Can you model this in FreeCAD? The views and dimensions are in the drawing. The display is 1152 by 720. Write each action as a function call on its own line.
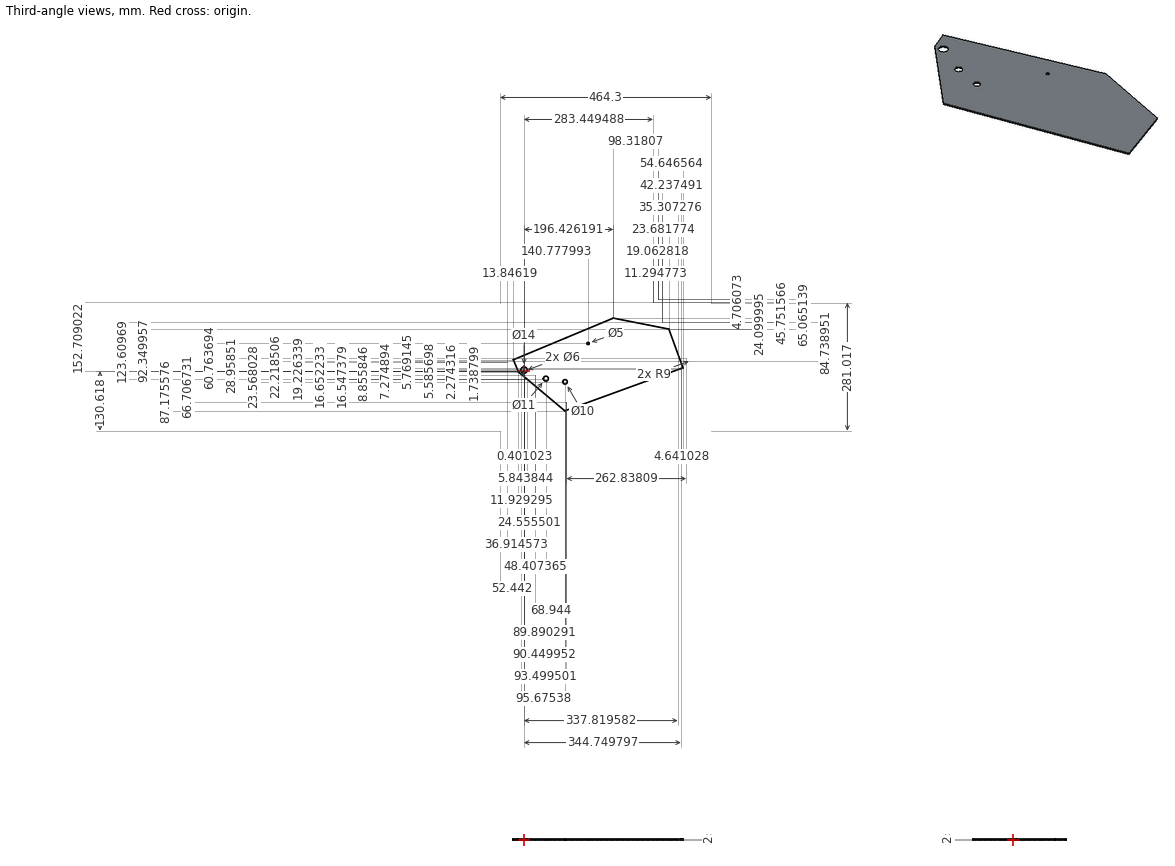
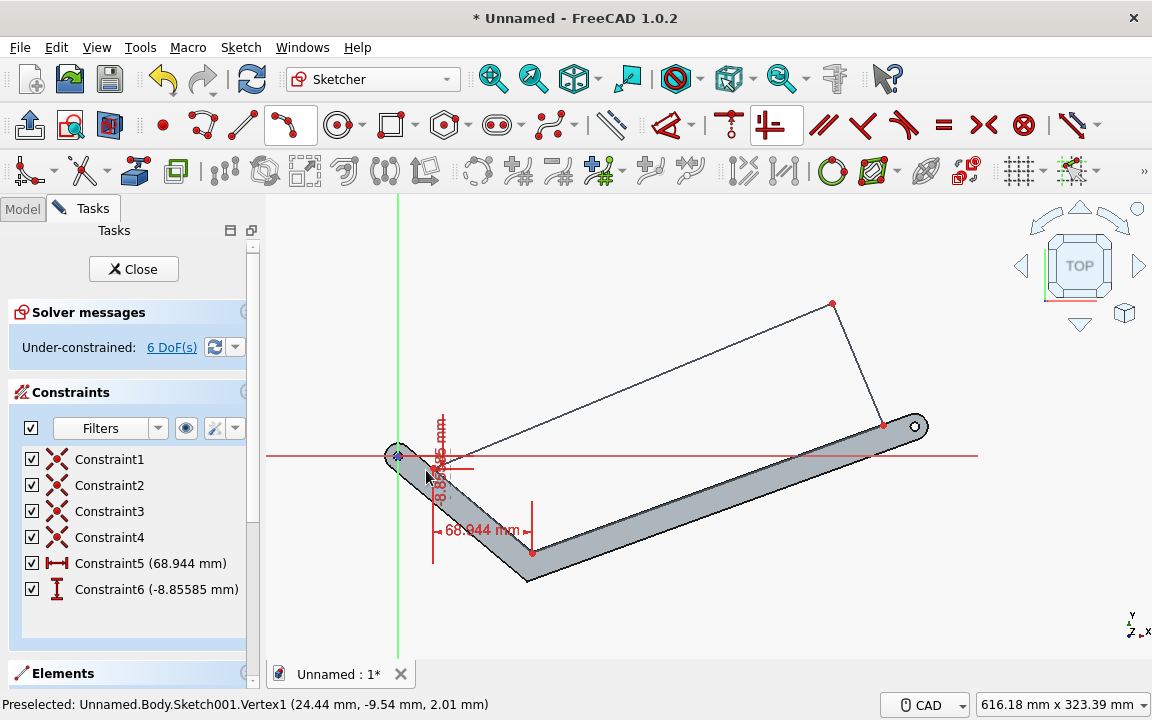
click(433, 469)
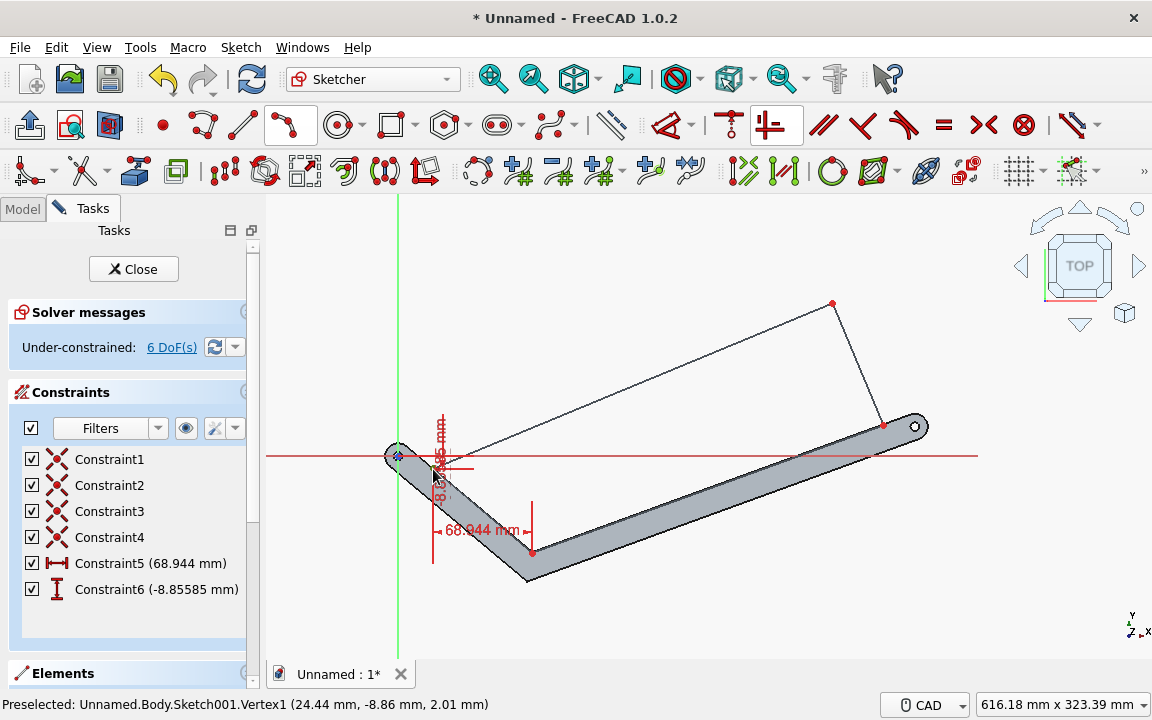
key(l)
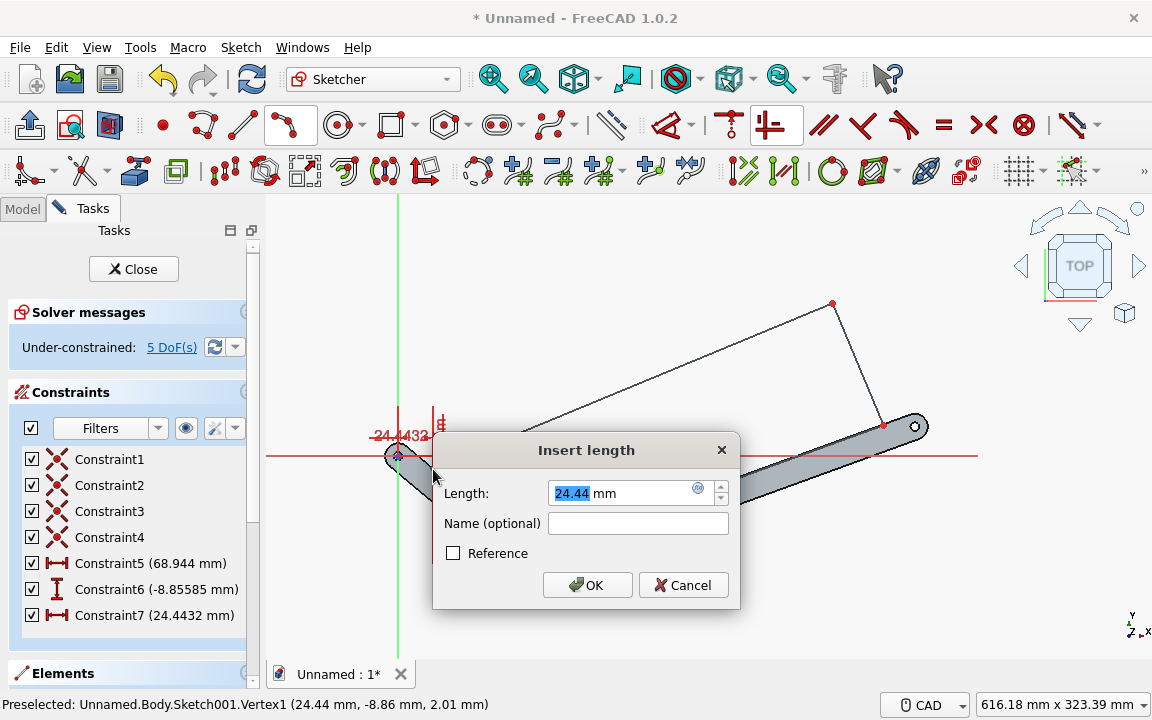
text(24.555501)
key(Return)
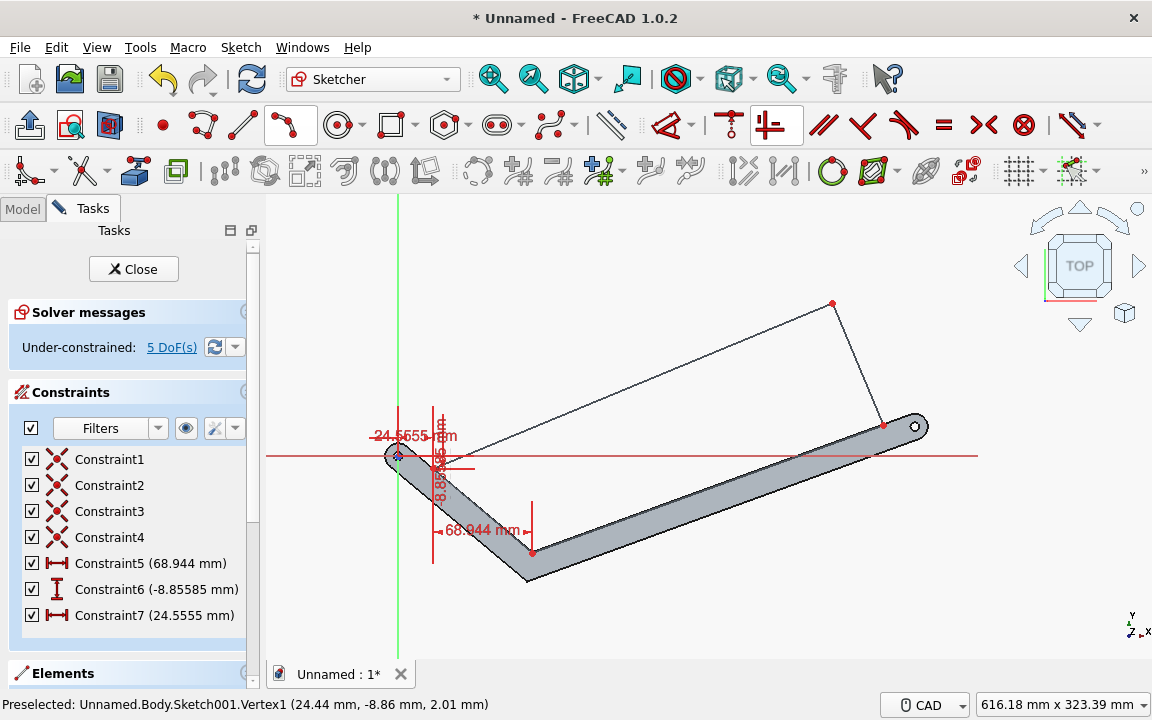
click(532, 553)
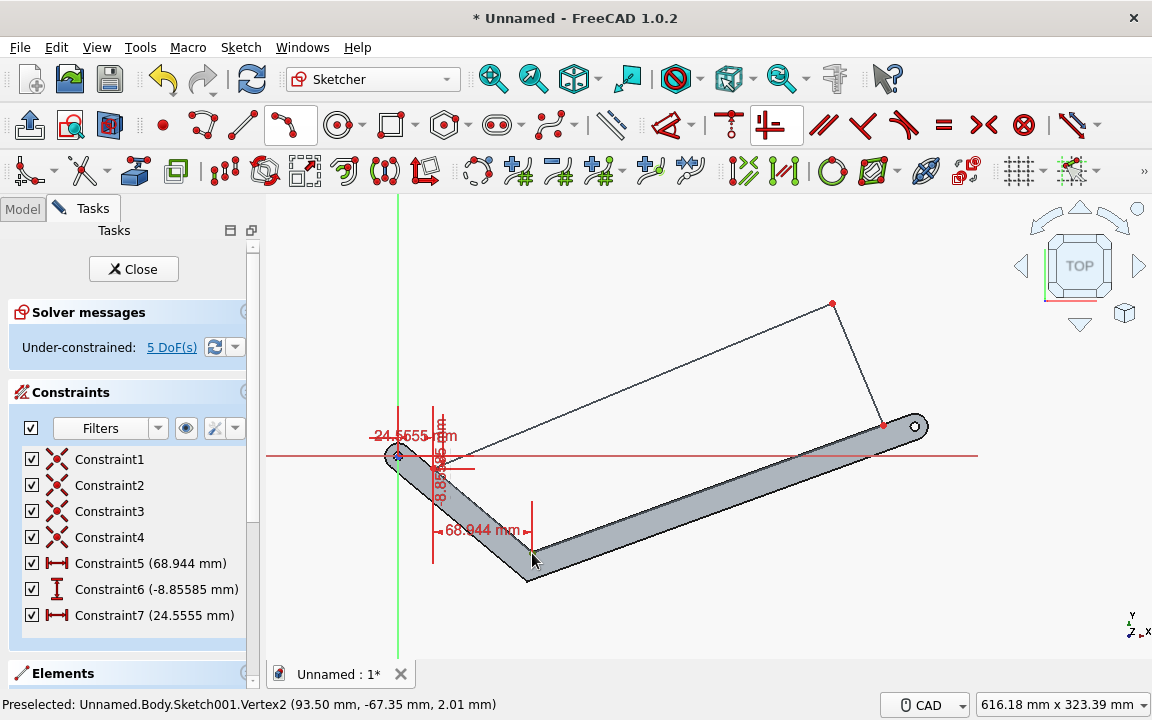
key(i)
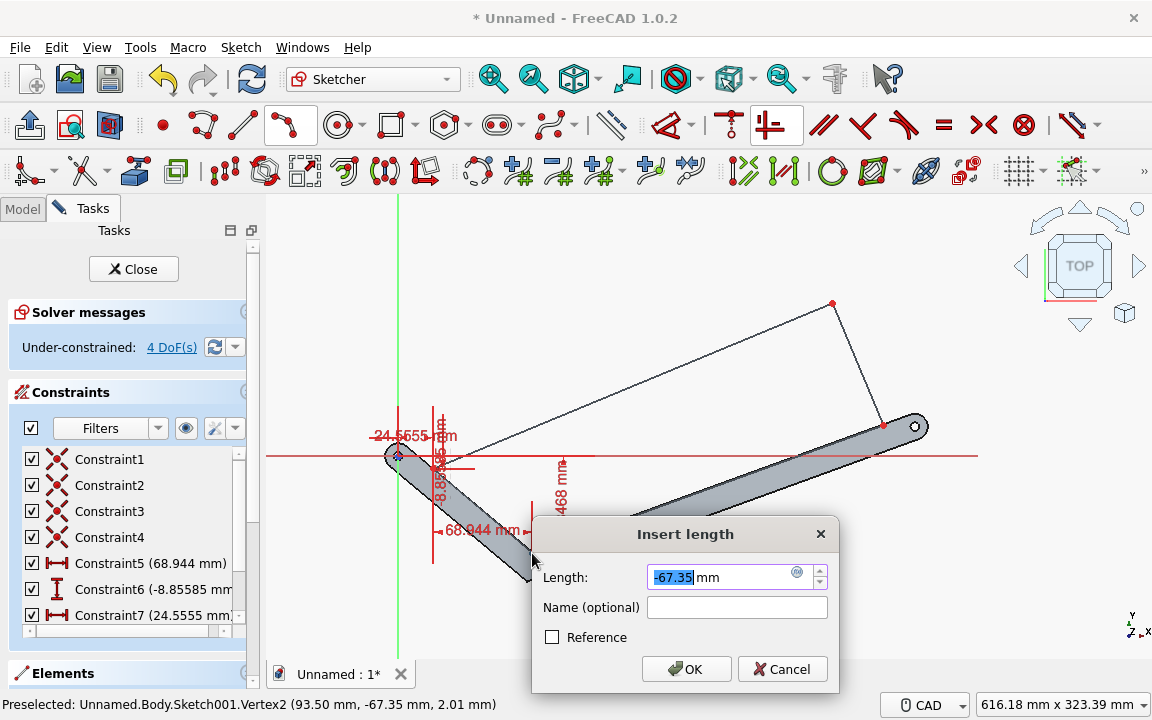
text(-66.706731)
key(Return)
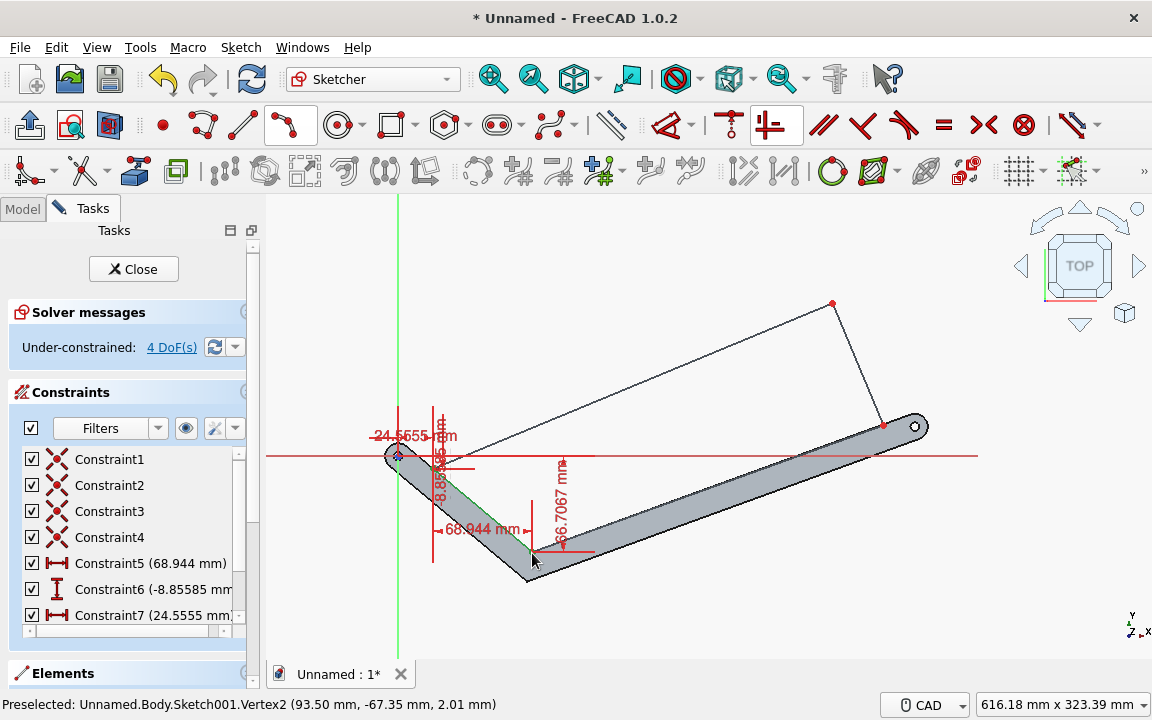
scroll(884, 425, up, 2)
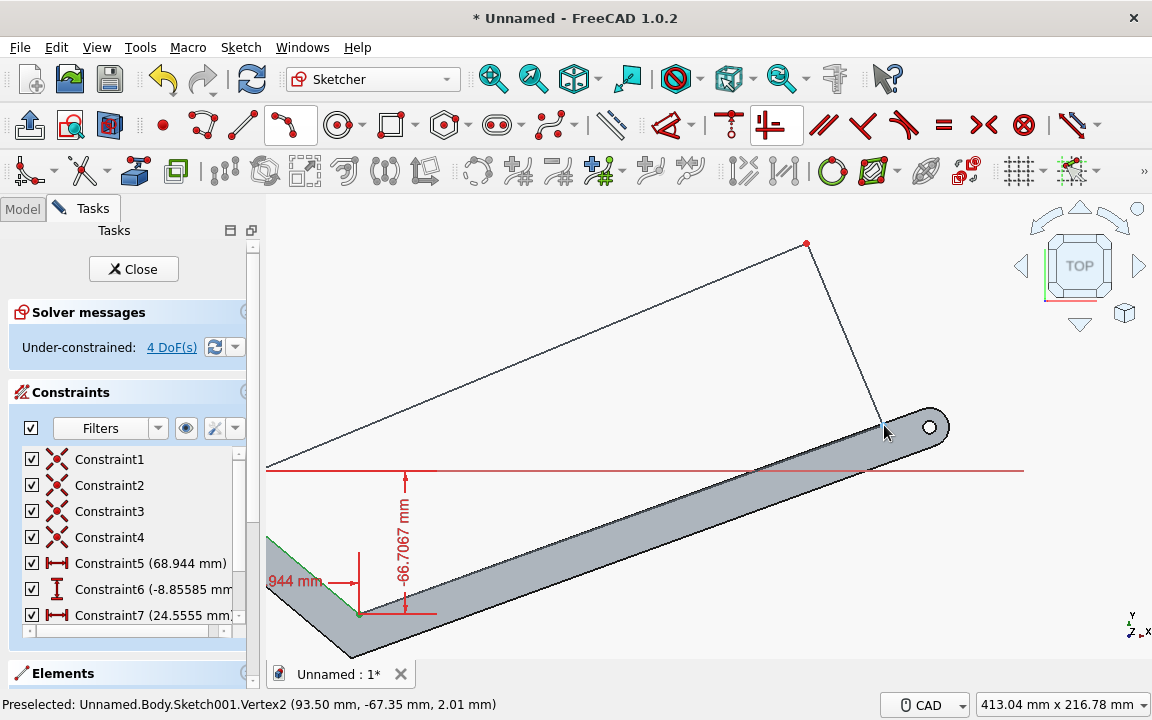
click(883, 425)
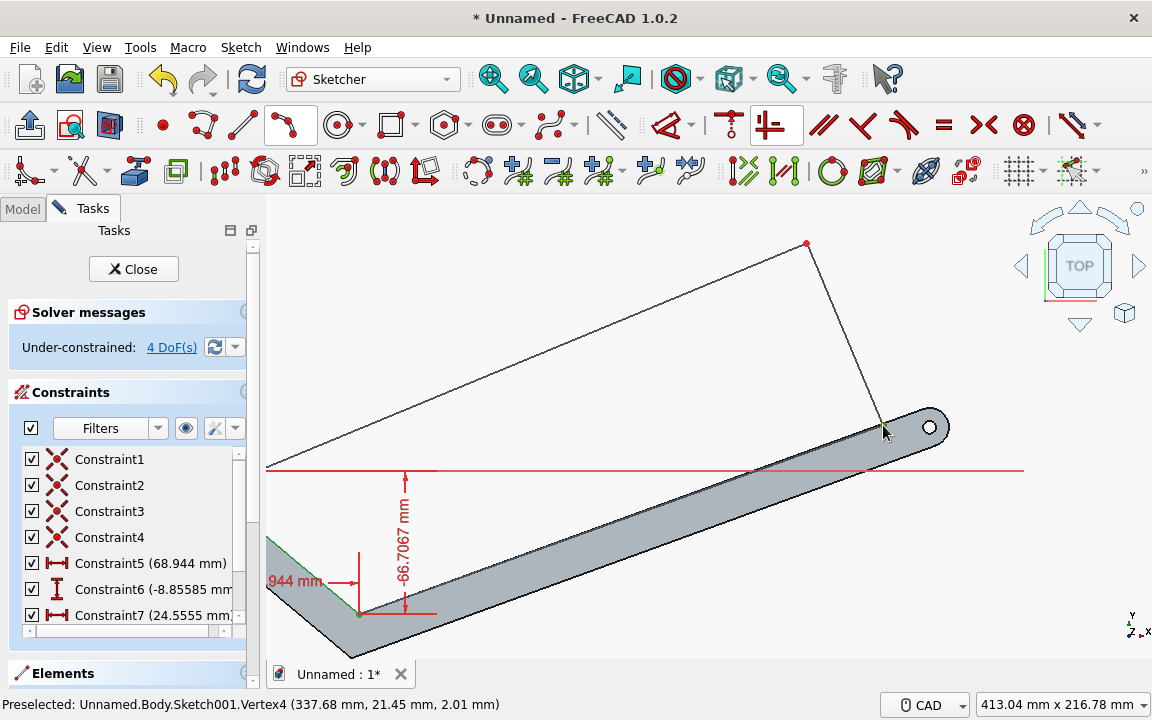
key(i)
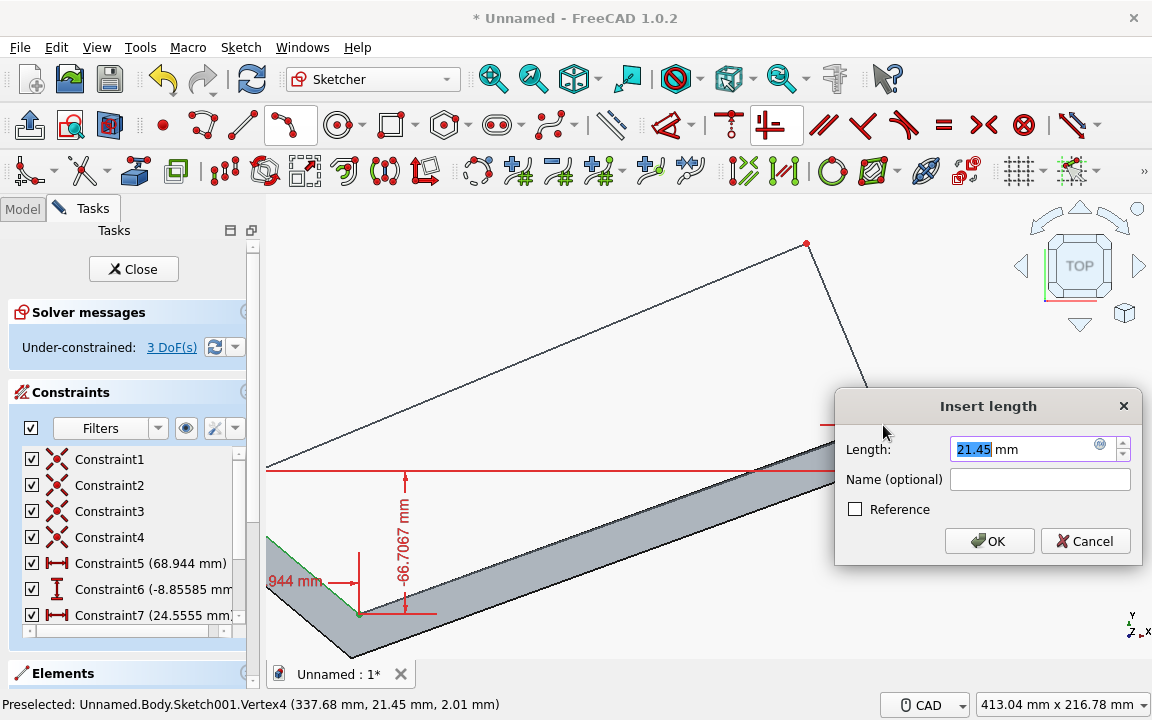
text(22.218506)
key(Return)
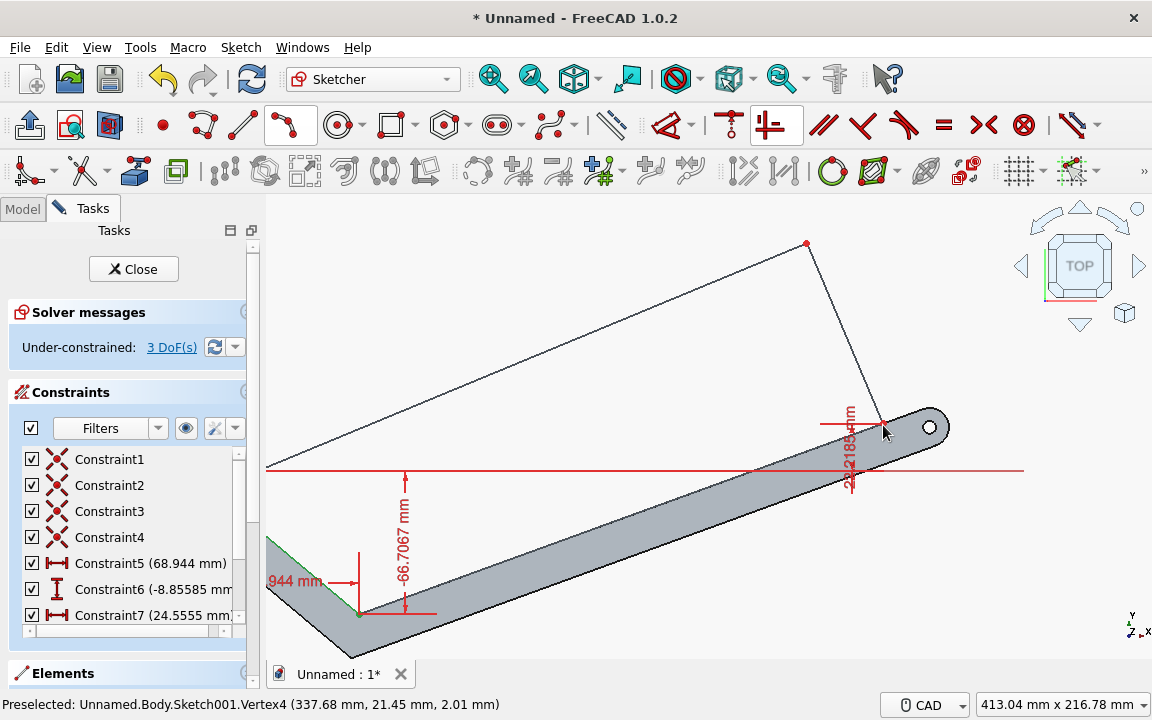
click(860, 369)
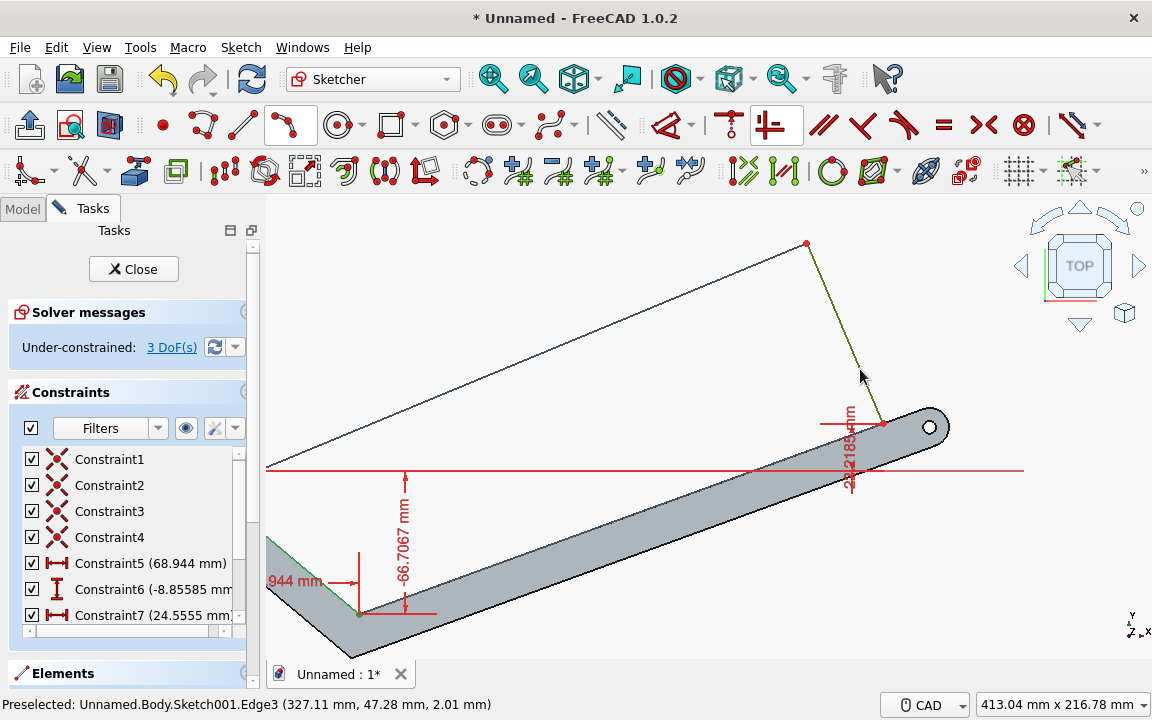
key(l)